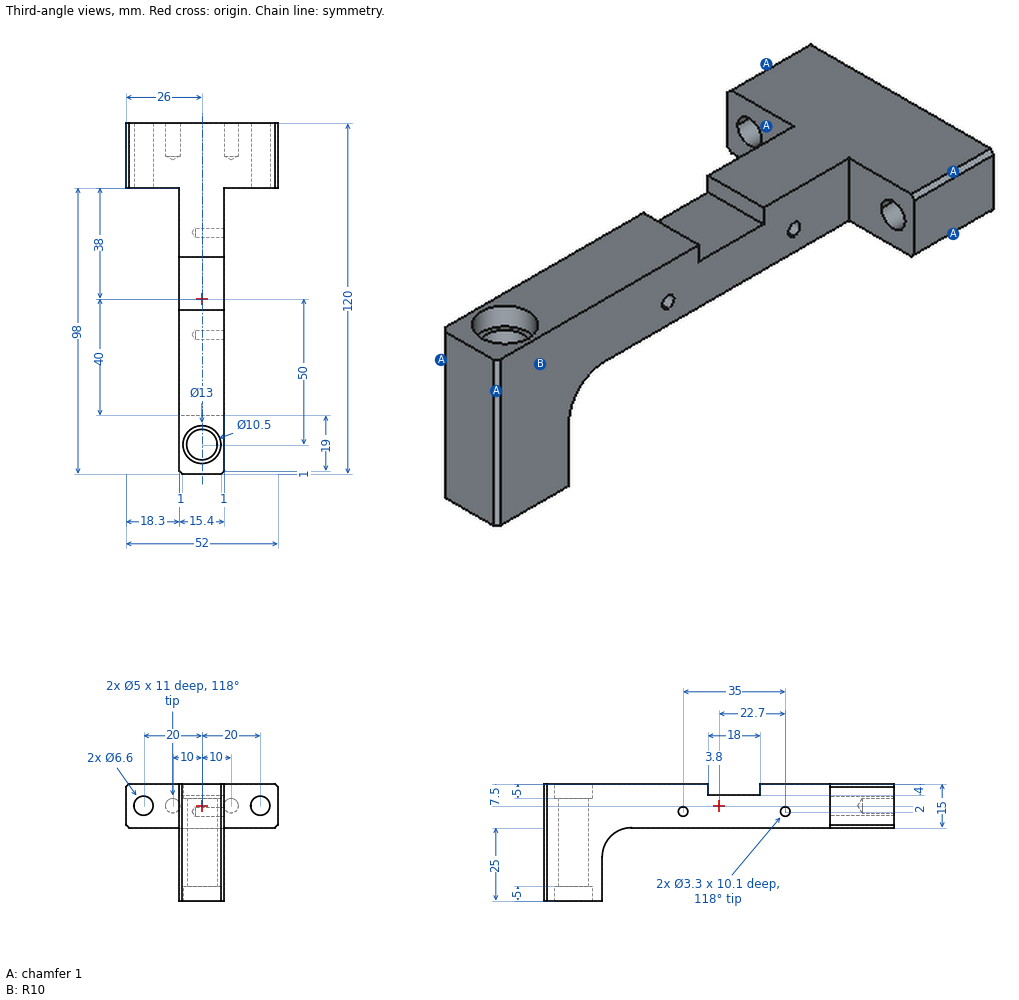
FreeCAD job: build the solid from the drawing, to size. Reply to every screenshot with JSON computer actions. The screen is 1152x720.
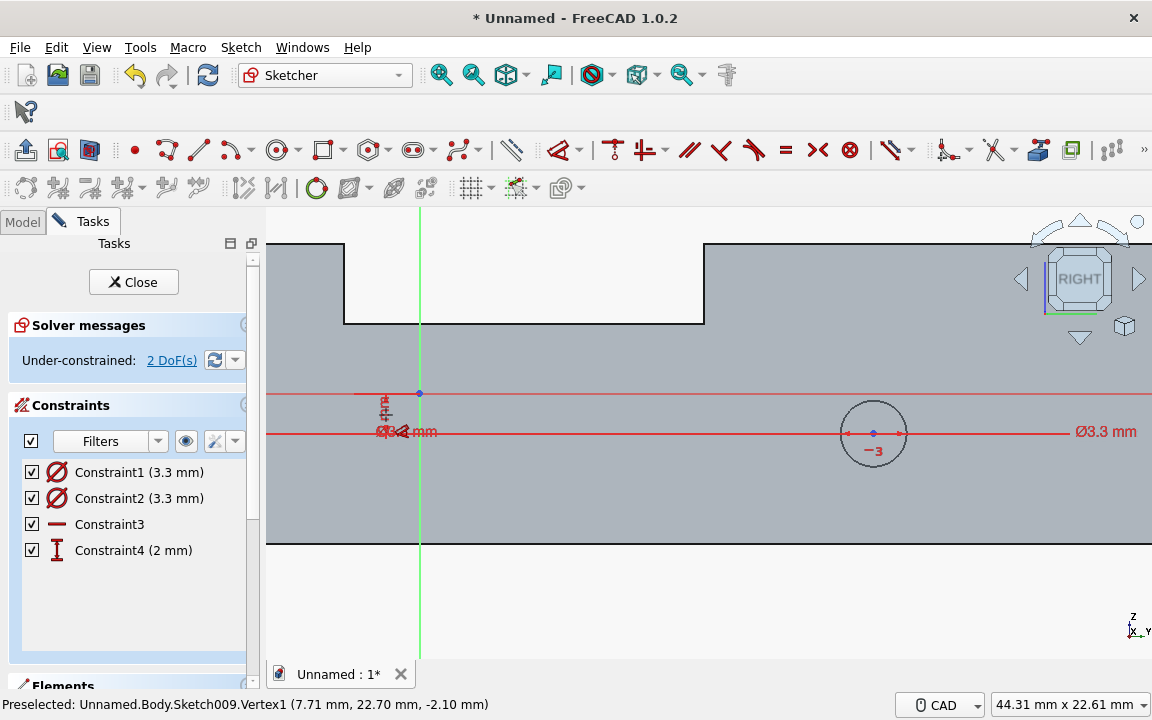
{"action": "left_click", "coordinate": [874, 434]}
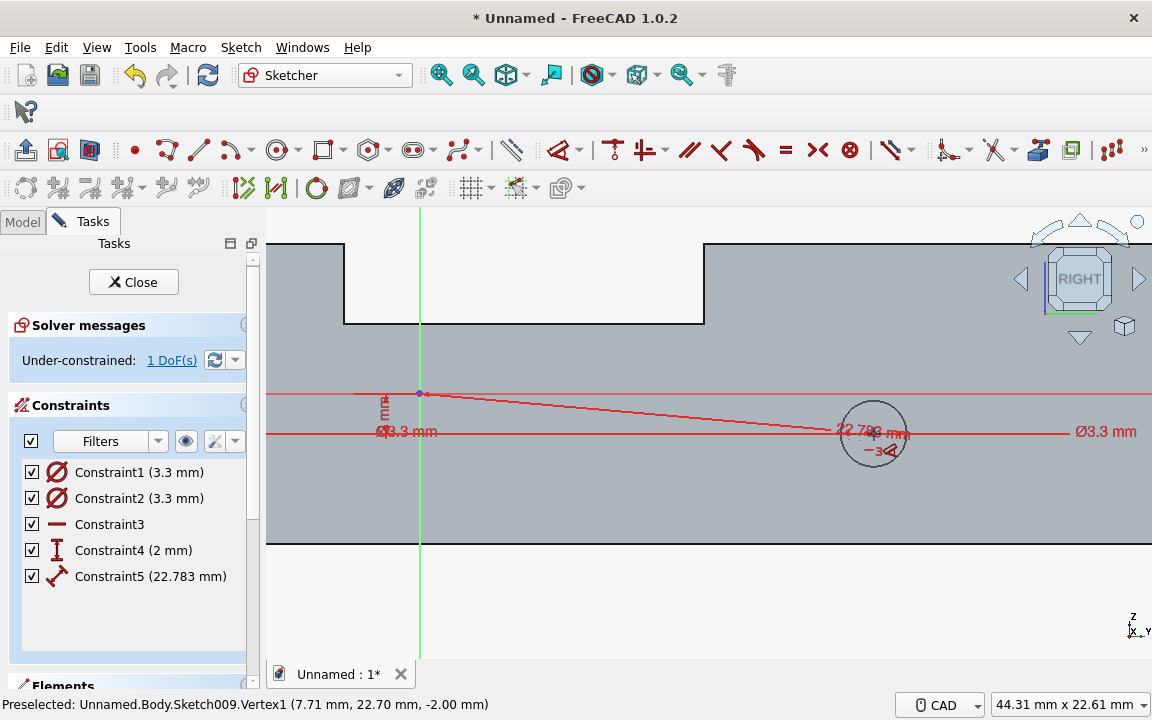
{"action": "scroll", "coordinate": [878, 439], "scroll_direction": "down", "scroll_amount": 2}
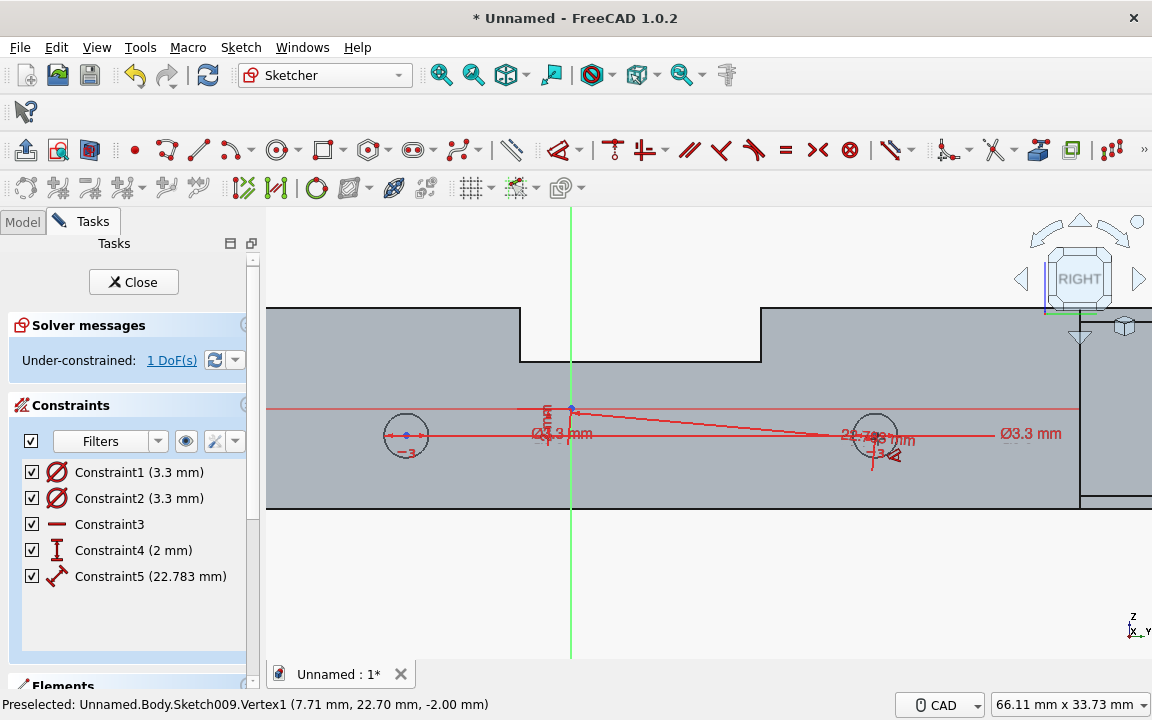
{"action": "left_click", "coordinate": [406, 436]}
{"action": "left_click", "coordinate": [641, 470]}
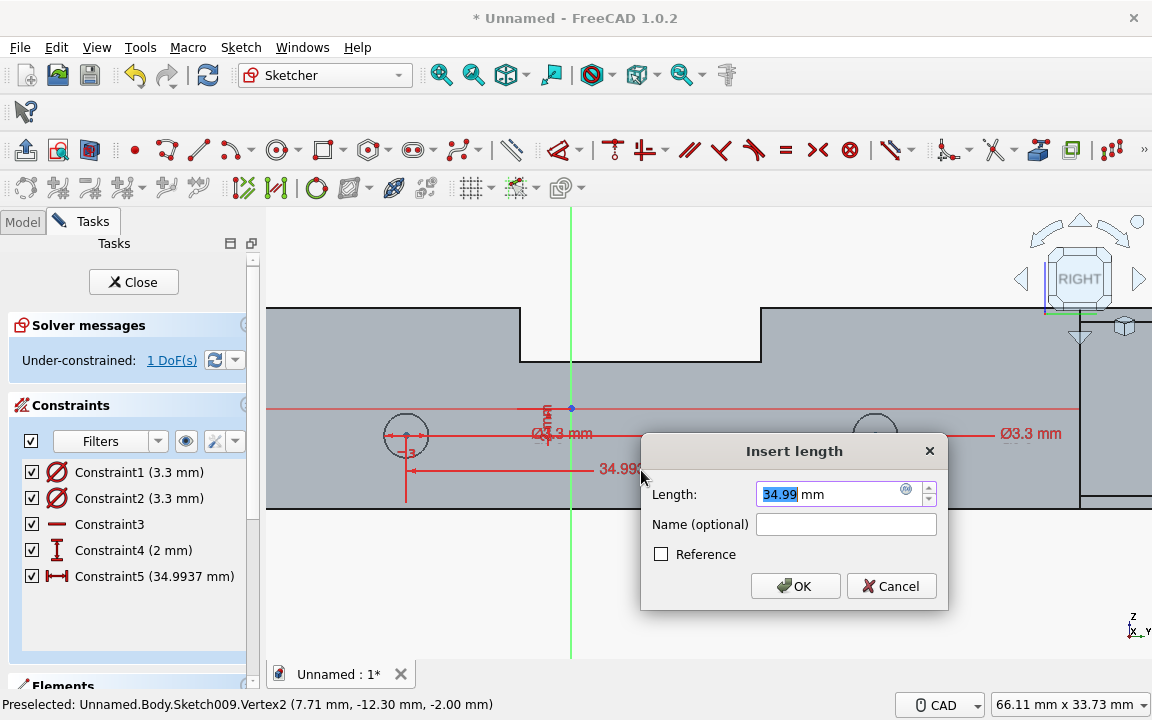
{"action": "type", "text": "35"}
{"action": "key", "text": "Return"}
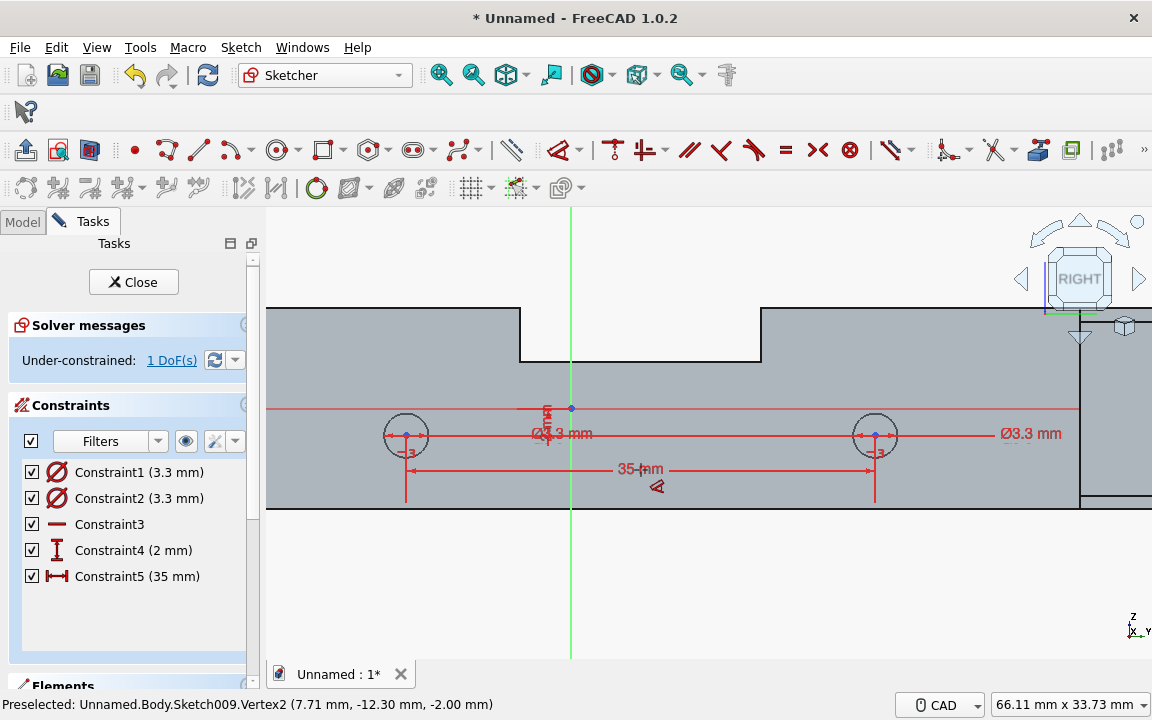
{"action": "left_click", "coordinate": [875, 436]}
{"action": "left_click", "coordinate": [723, 375]}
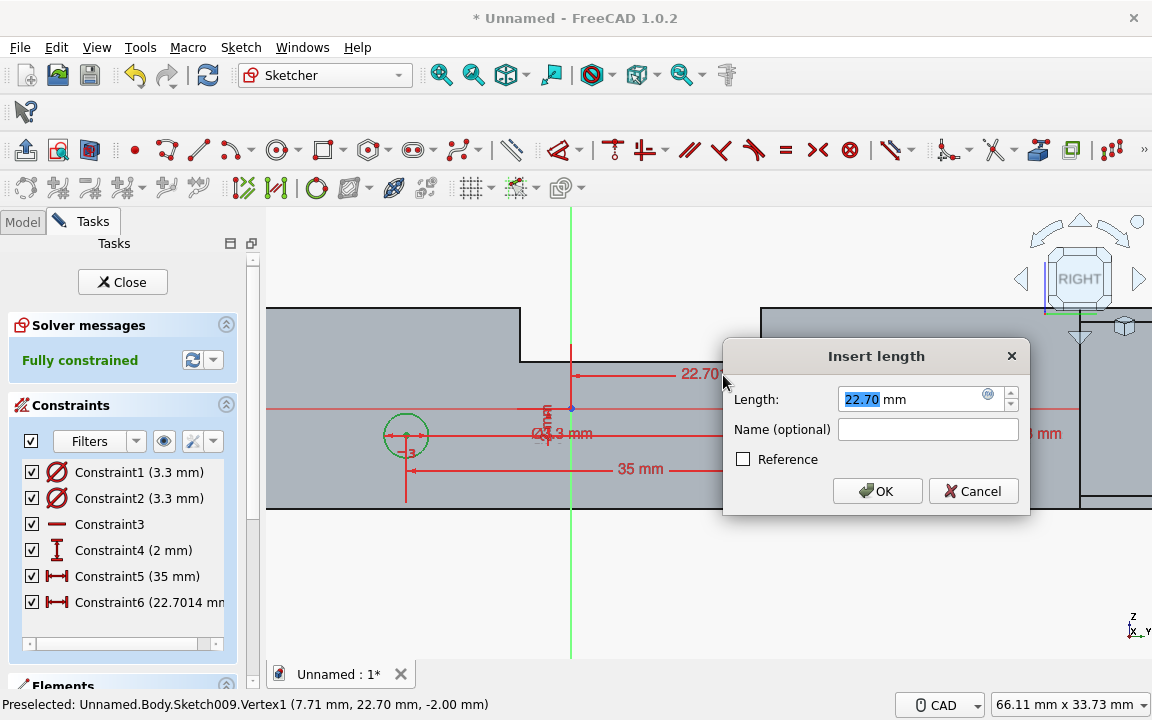
{"action": "type", "text": "22.7"}
{"action": "key", "text": "Return"}
{"action": "key", "text": "Escape"}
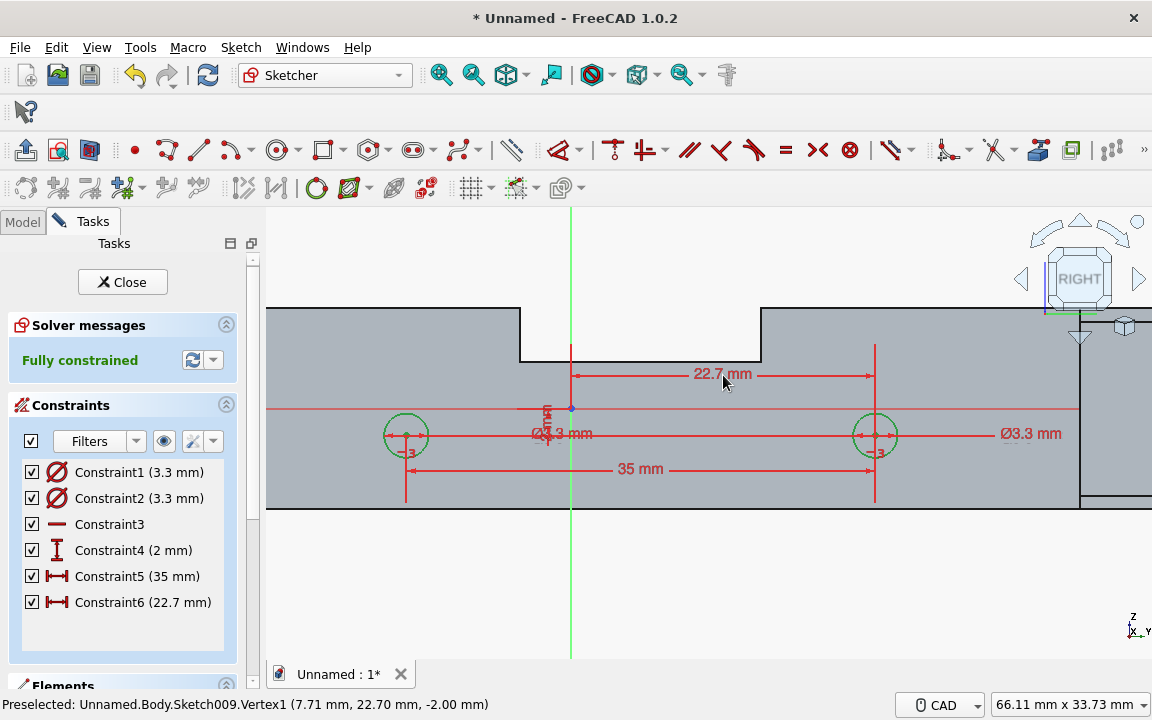
{"action": "left_click", "coordinate": [123, 282]}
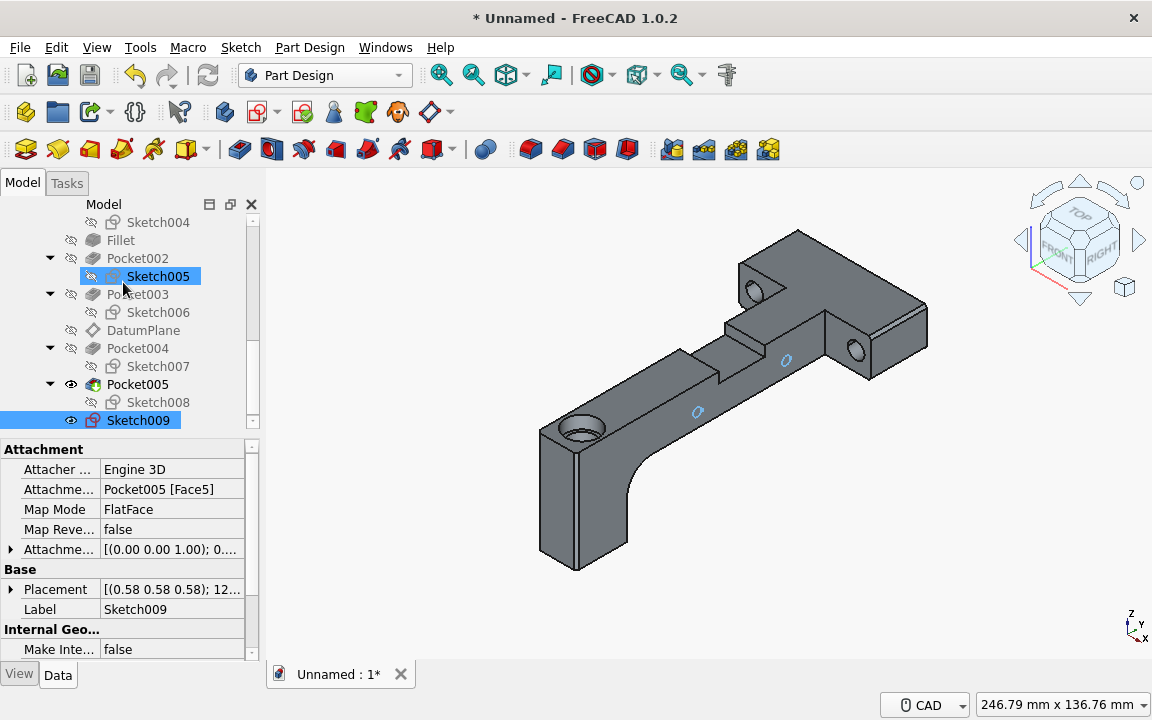
{"action": "left_click", "coordinate": [272, 150]}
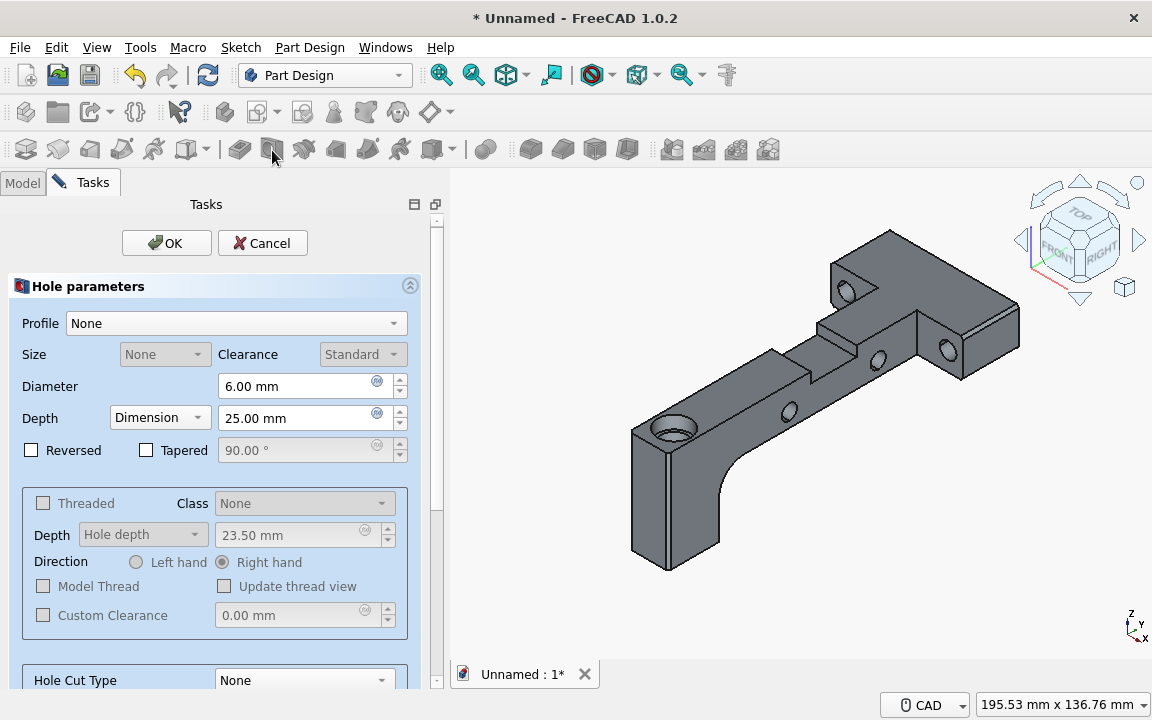
{"action": "triple_click", "coordinate": [305, 386]}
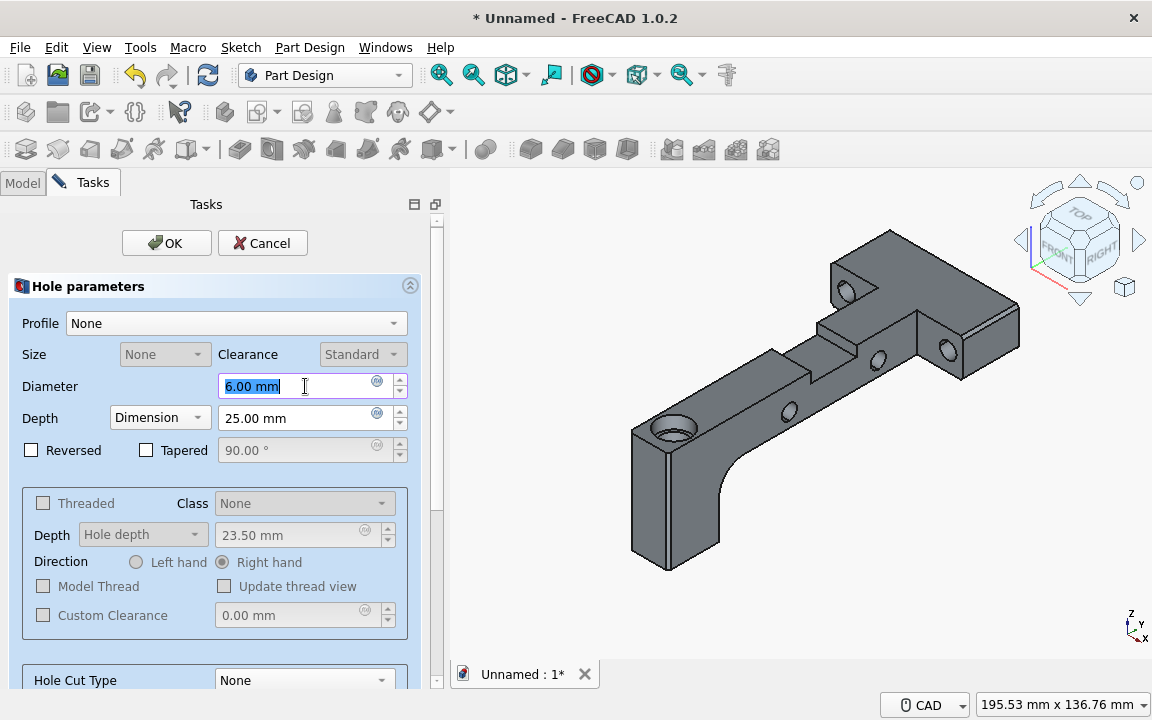
{"action": "type", "text": "3.3"}
{"action": "key", "text": "Tab"}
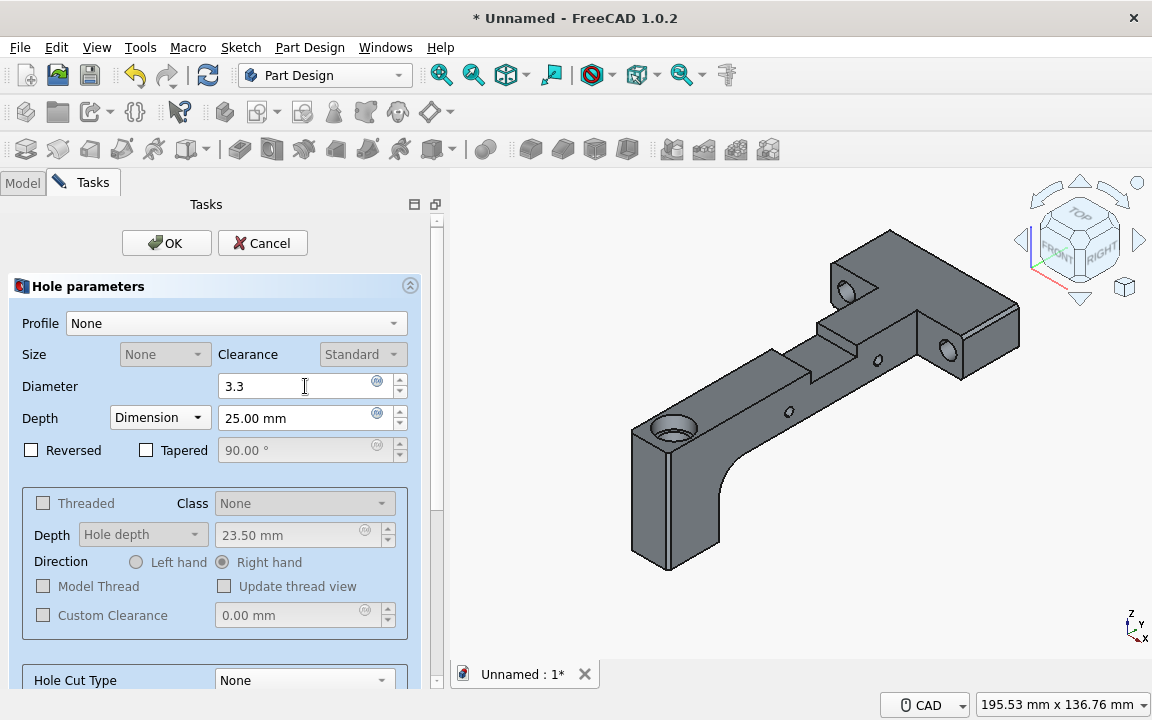
{"action": "triple_click", "coordinate": [305, 418]}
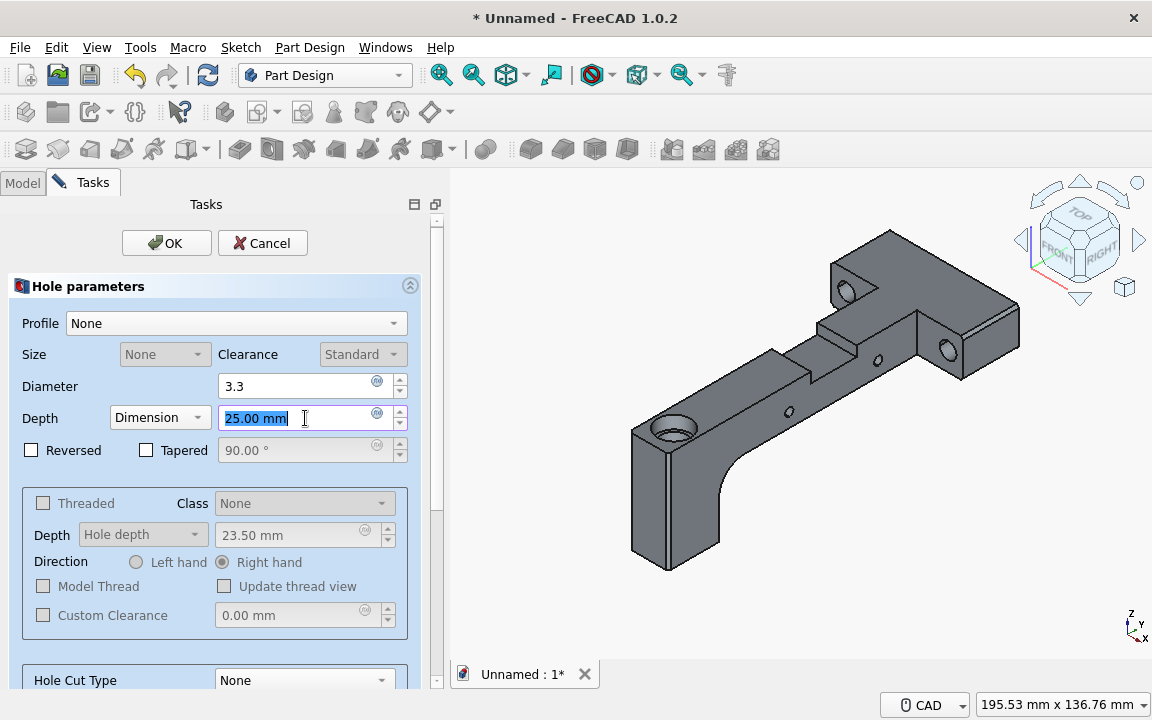
{"action": "type", "text": "10.1"}
{"action": "key", "text": "Tab"}